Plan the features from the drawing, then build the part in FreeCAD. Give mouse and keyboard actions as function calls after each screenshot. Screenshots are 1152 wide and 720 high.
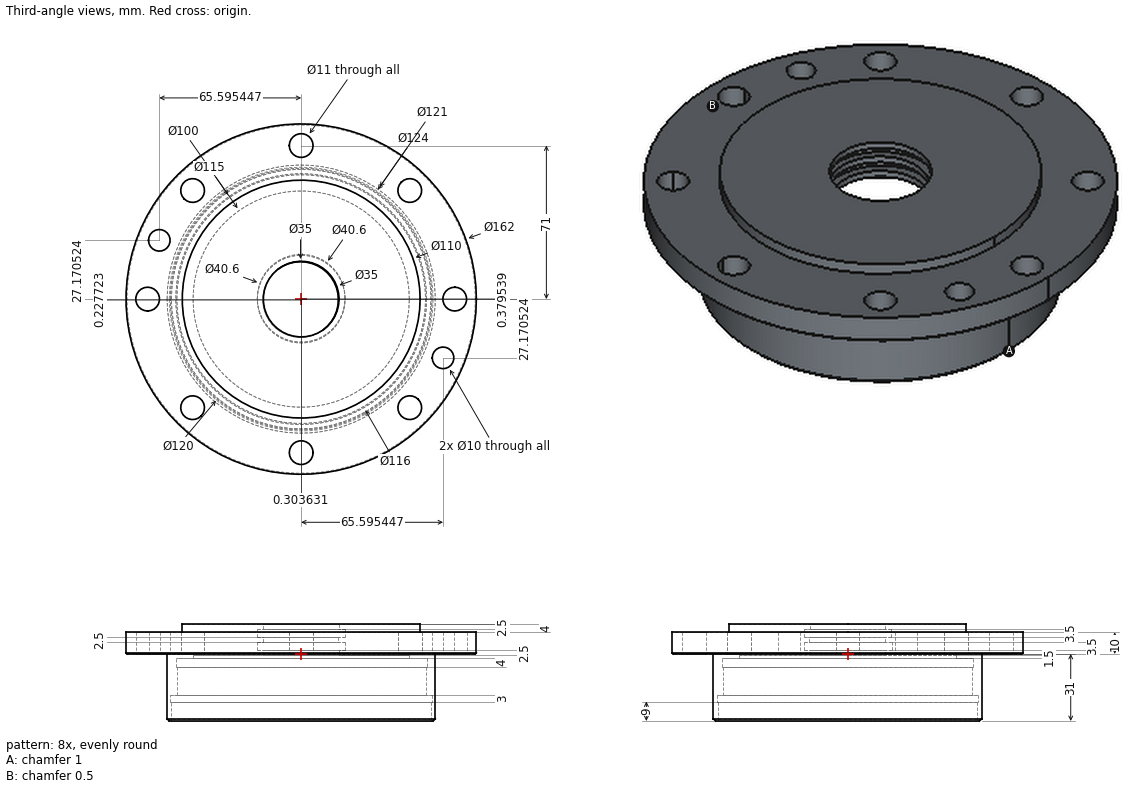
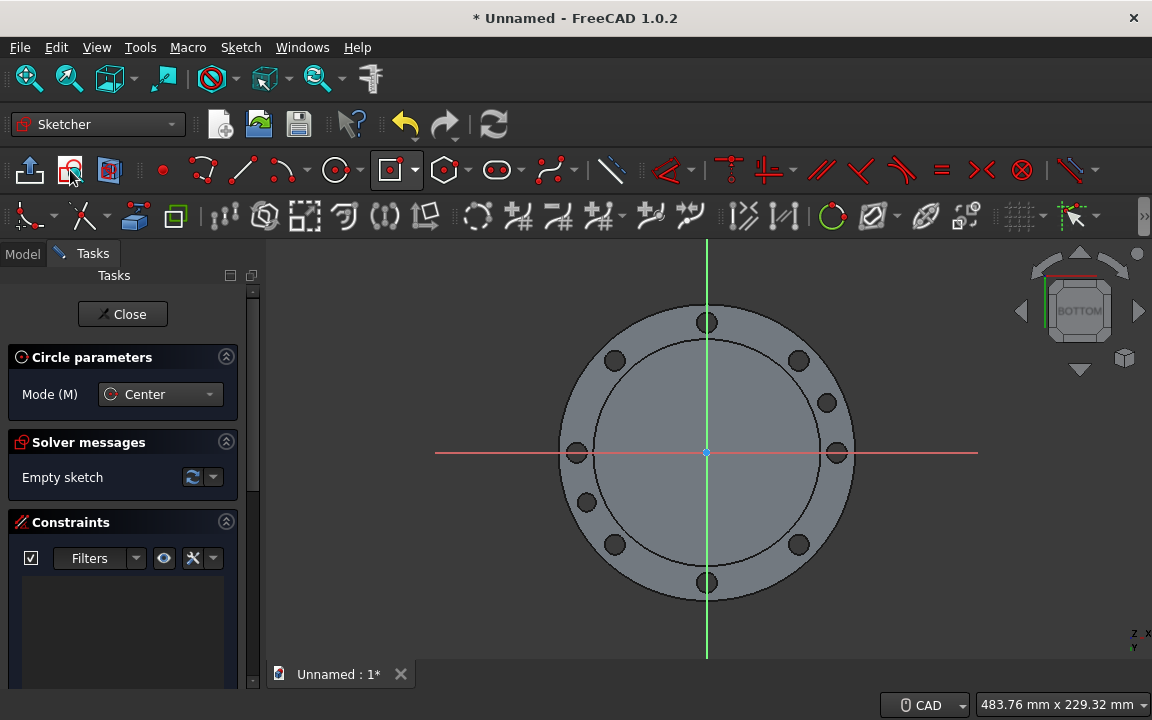
click(707, 453)
click(785, 375)
key(Escape)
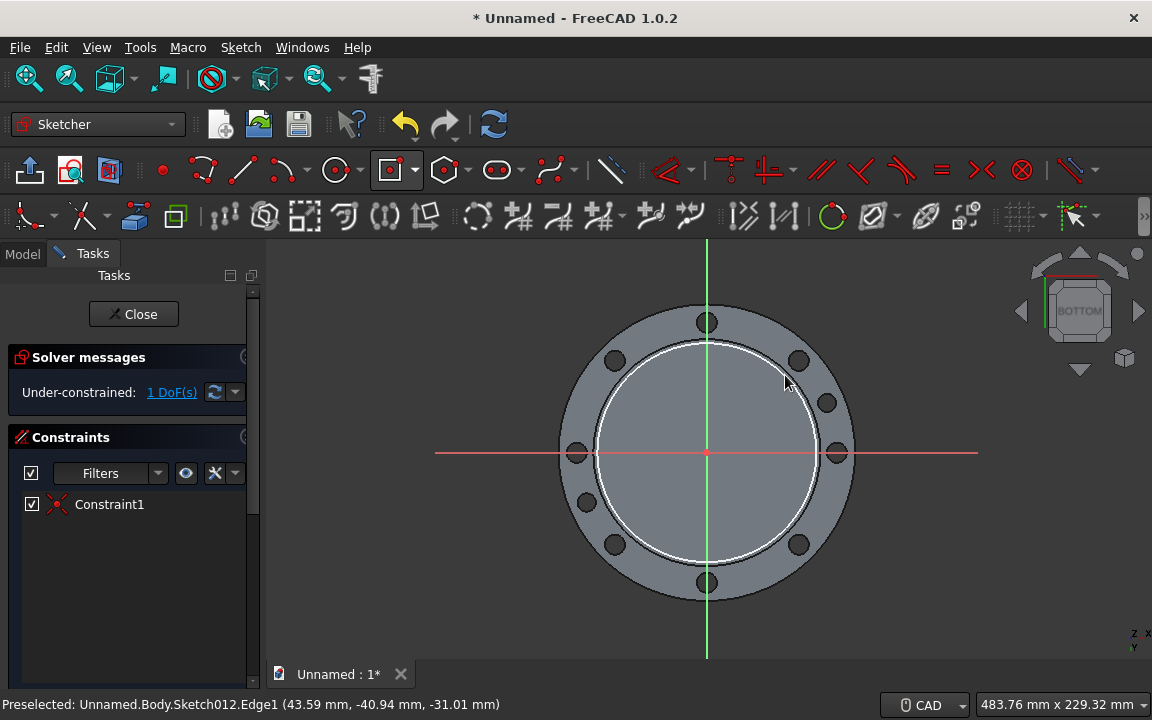
click(666, 170)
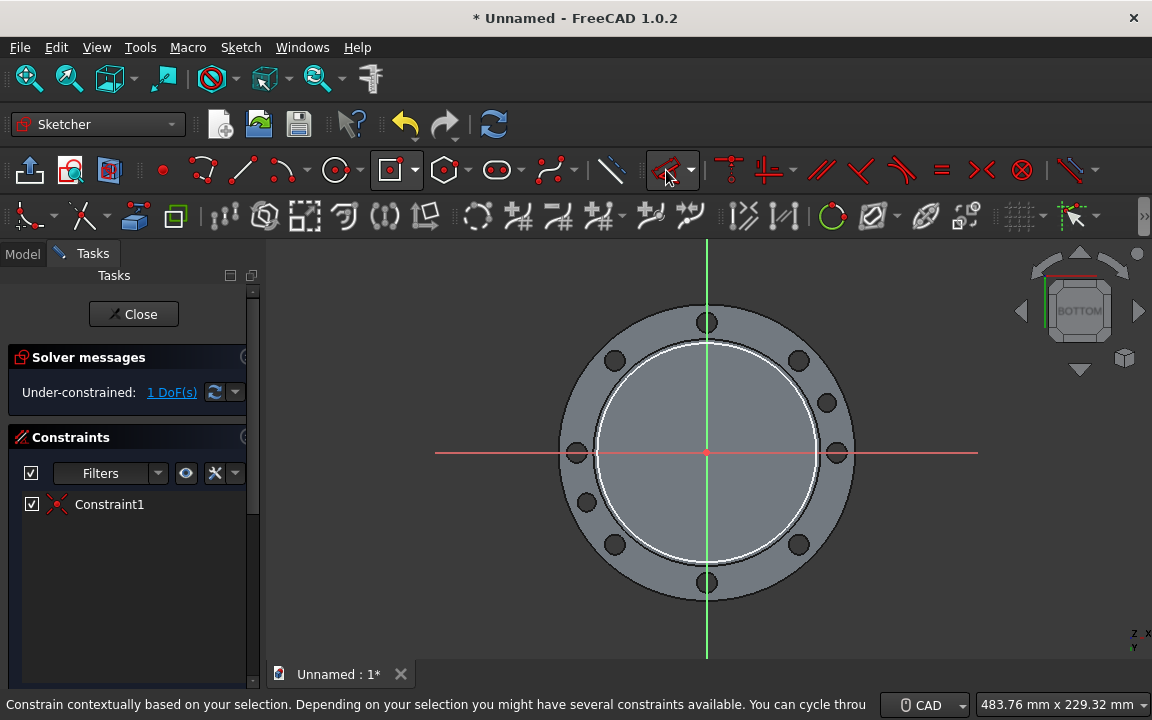
click(784, 375)
click(807, 352)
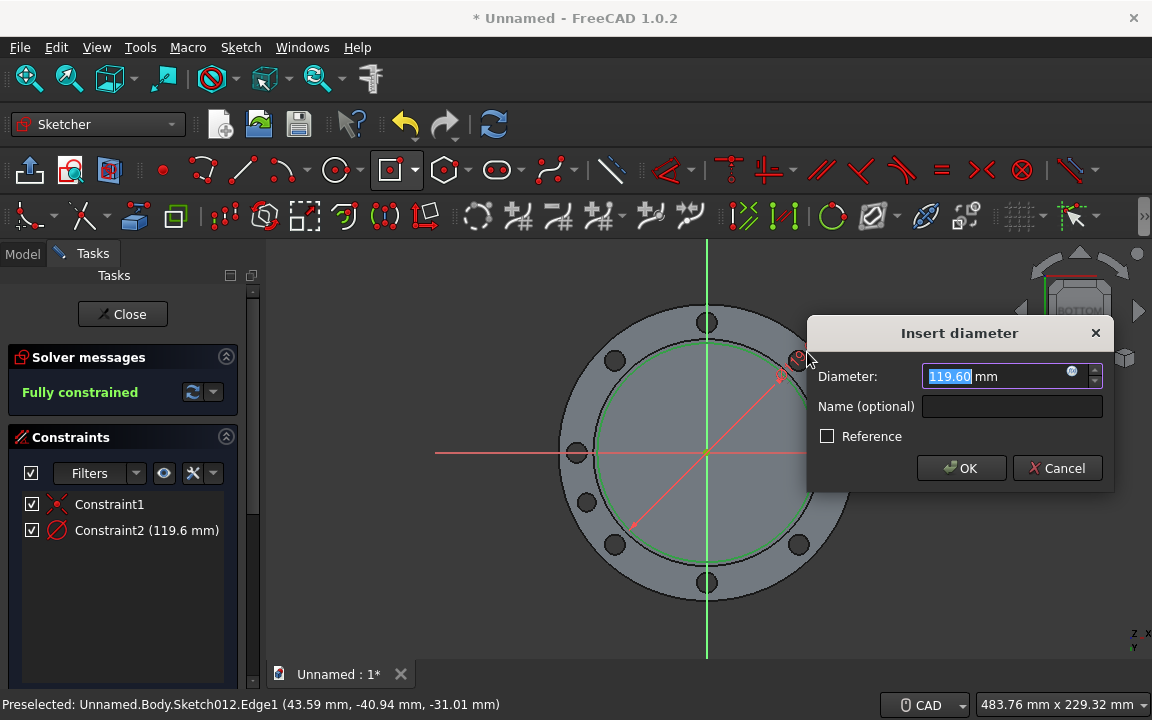
text(120)
key(Return)
key(Escape)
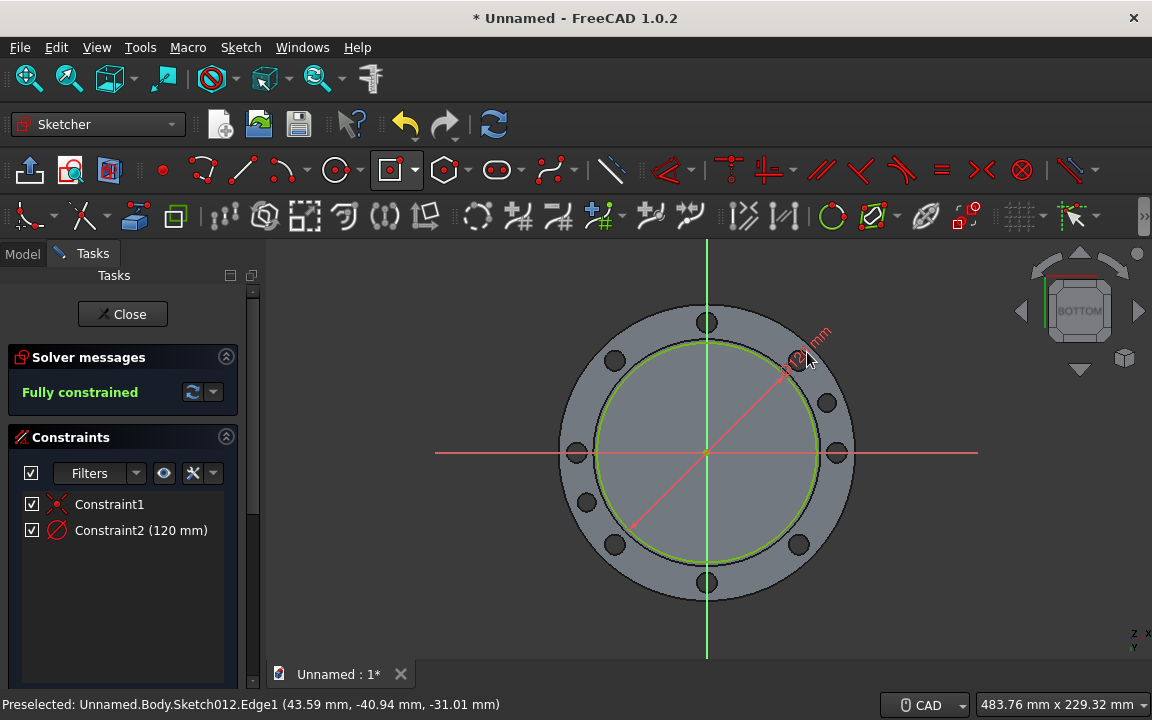
click(123, 314)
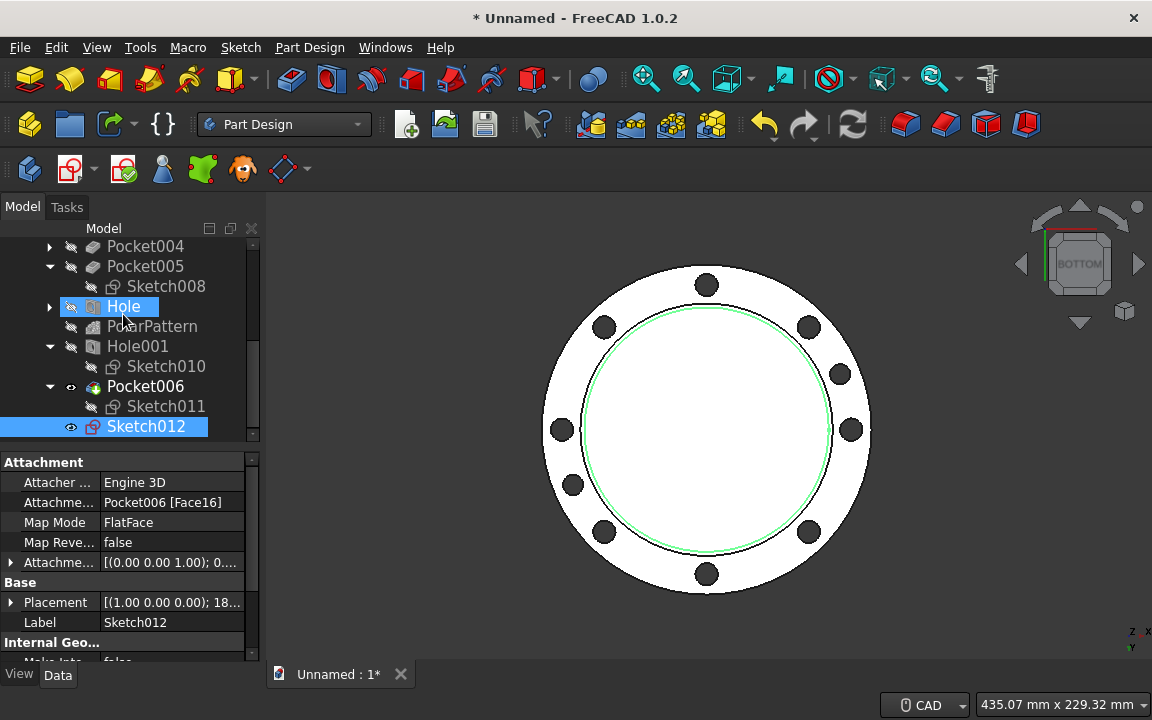
click(292, 80)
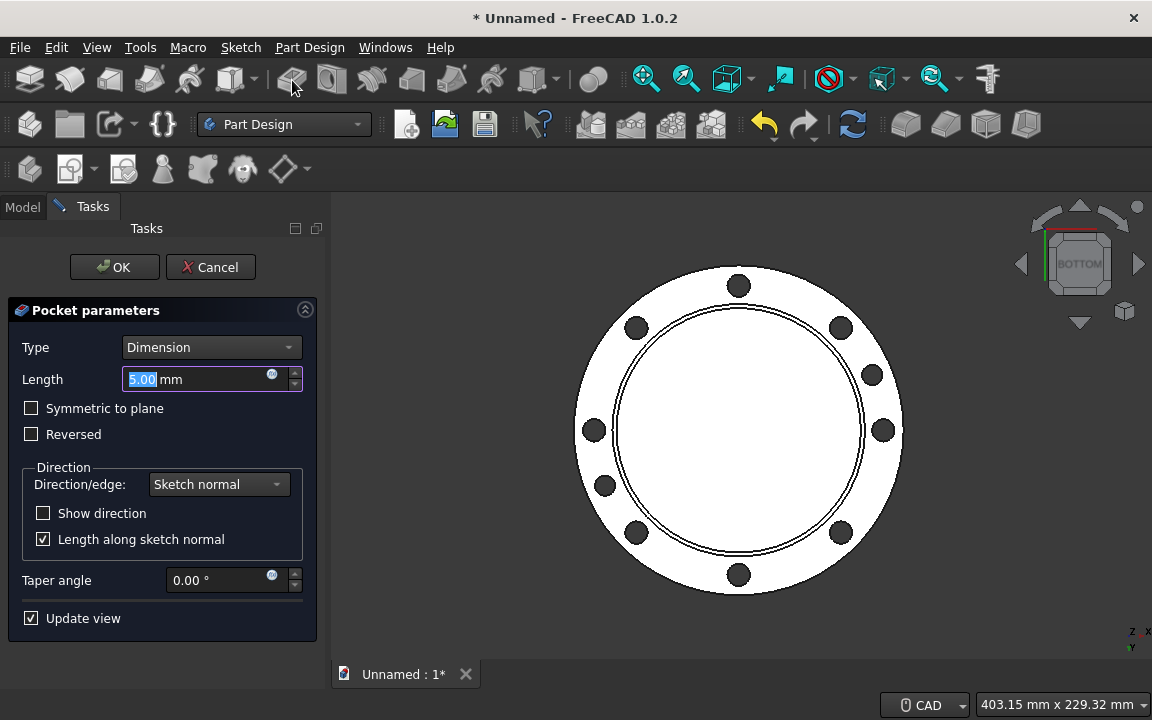
text(9)
key(Tab)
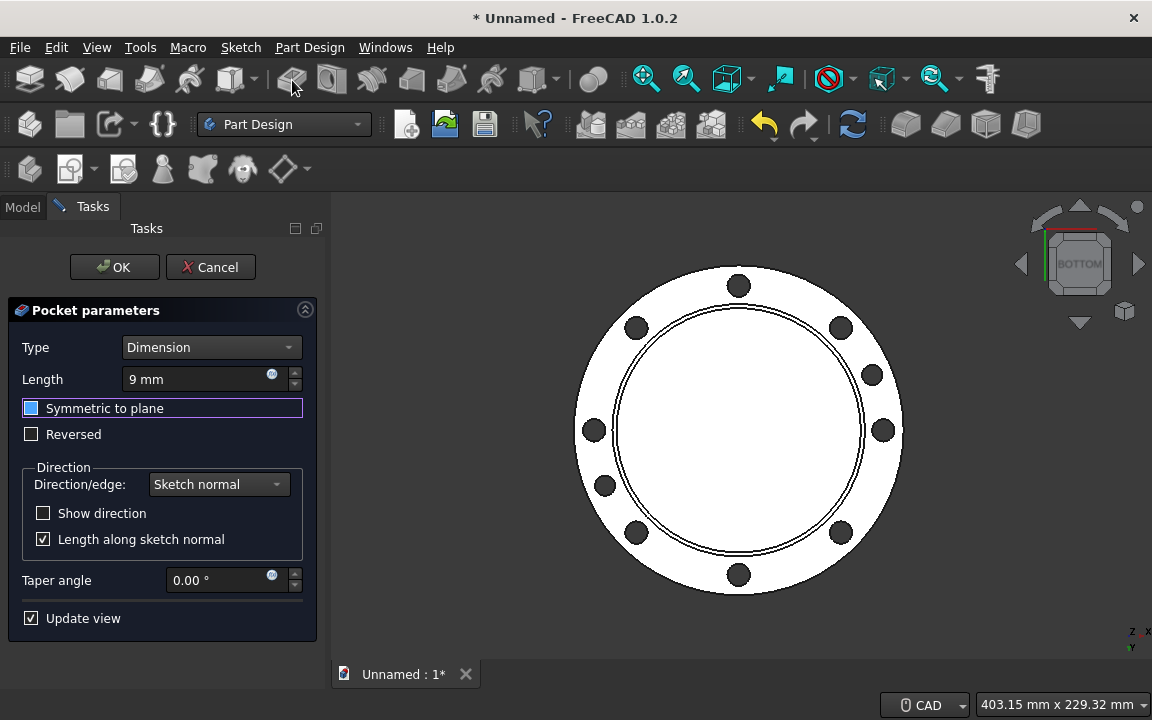
click(115, 267)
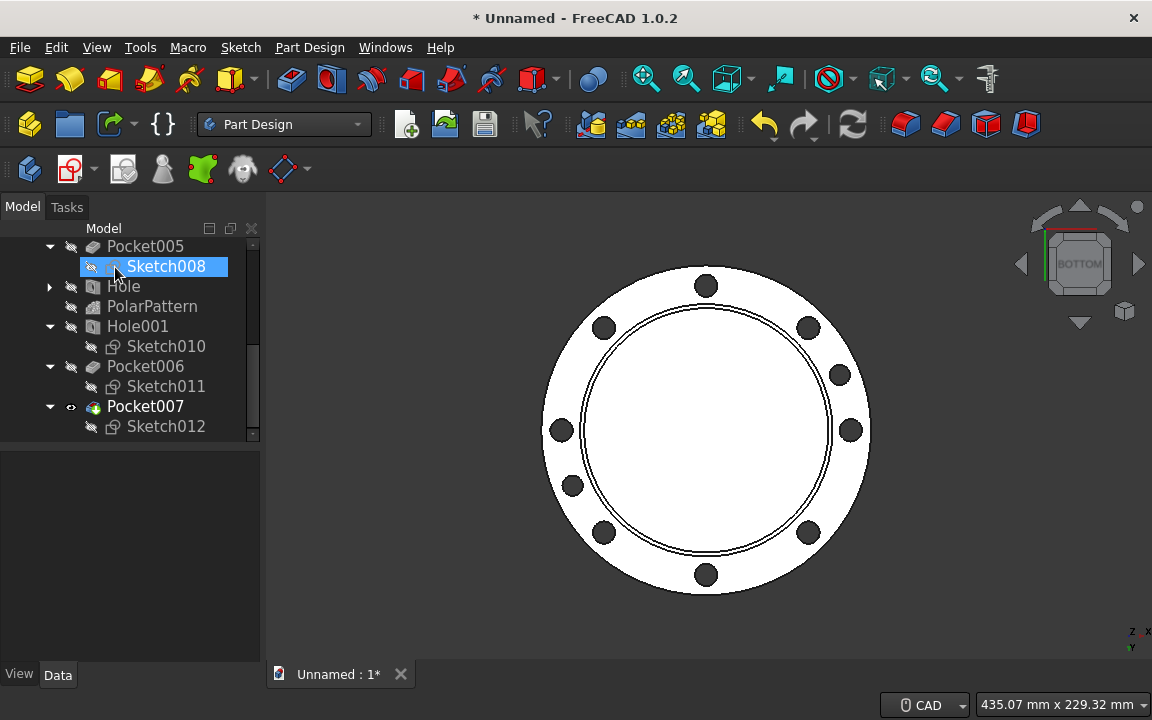
click(706, 429)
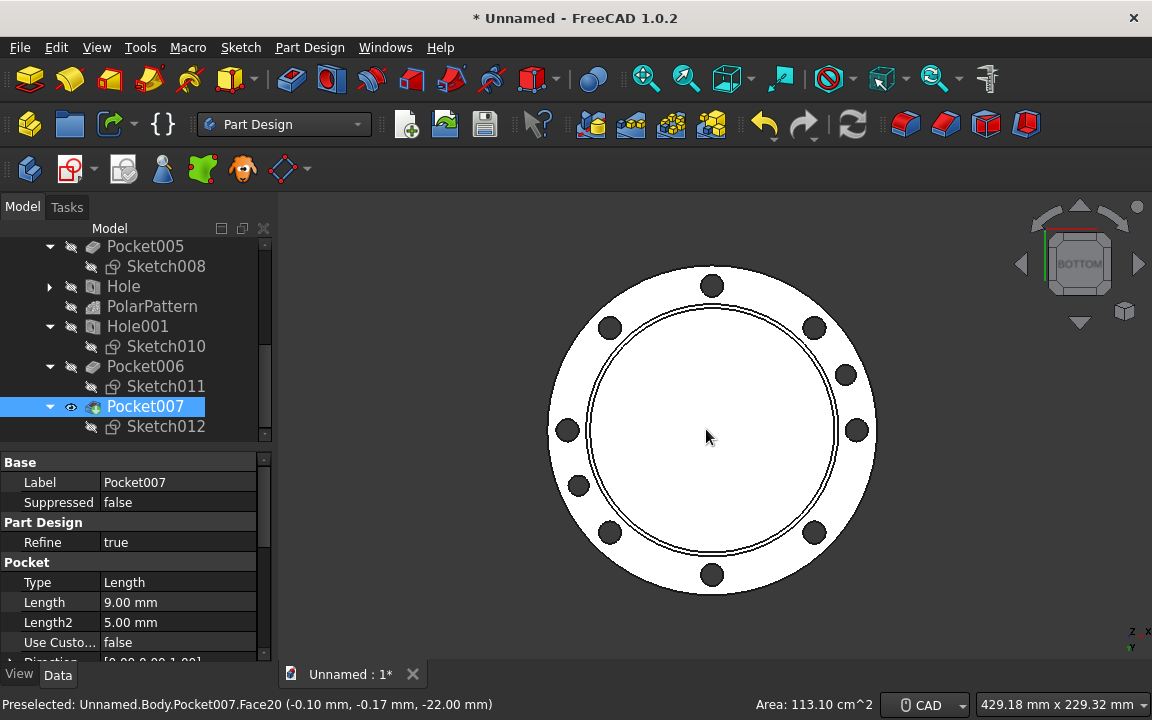
click(70, 170)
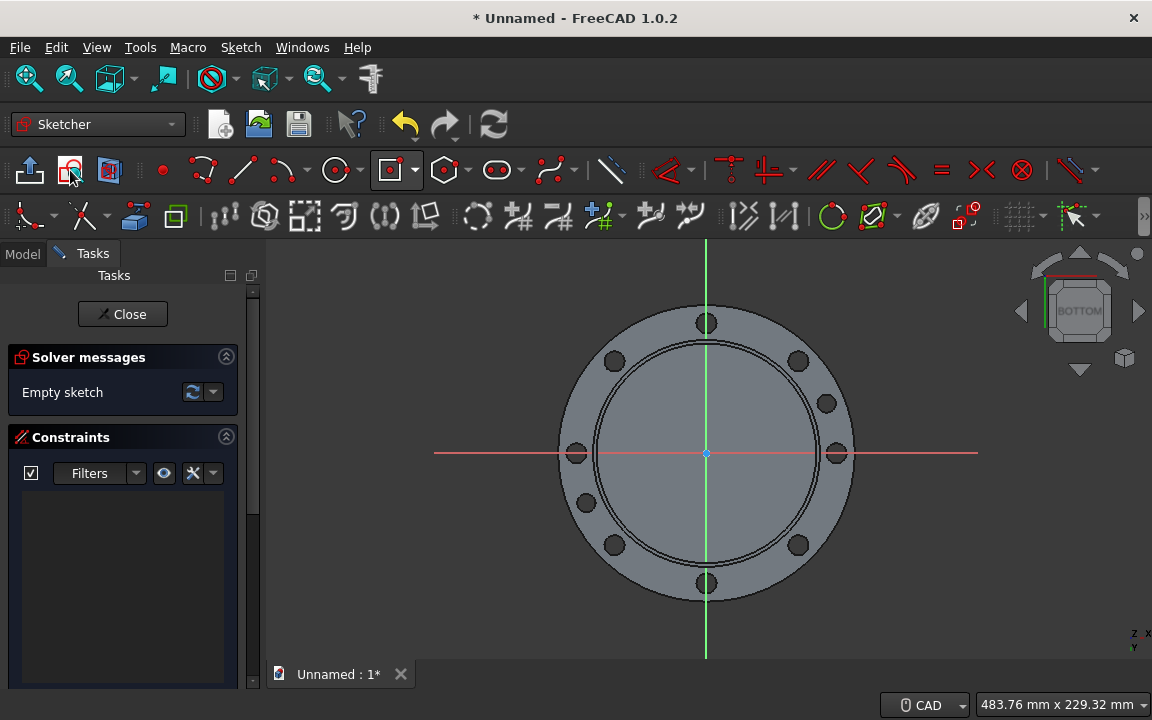
click(110, 170)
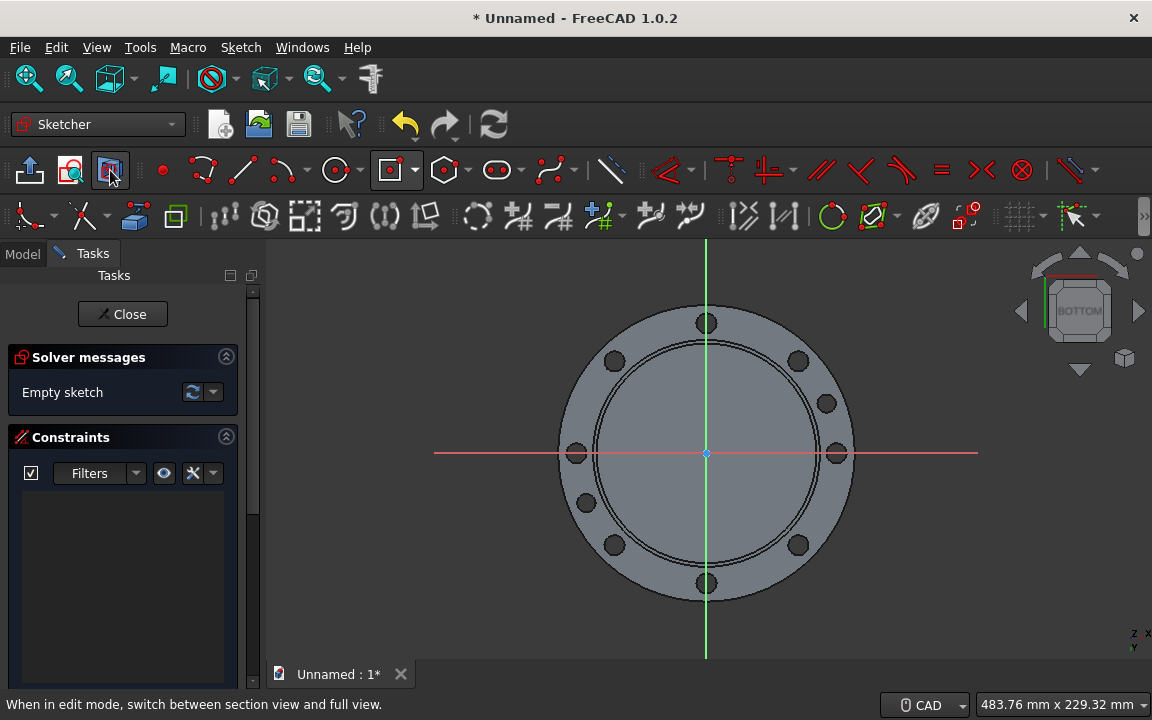
click(336, 170)